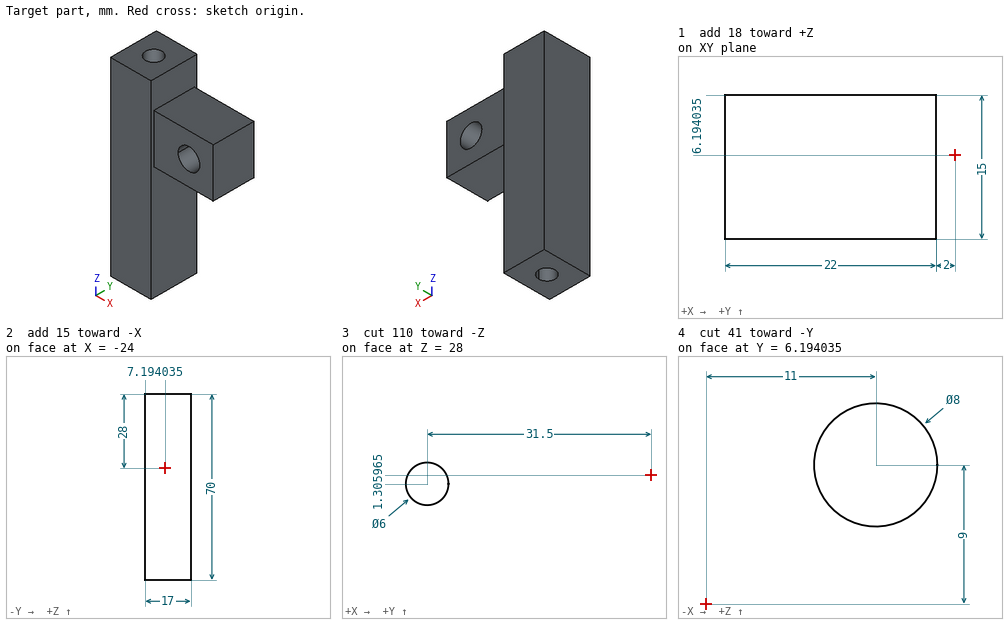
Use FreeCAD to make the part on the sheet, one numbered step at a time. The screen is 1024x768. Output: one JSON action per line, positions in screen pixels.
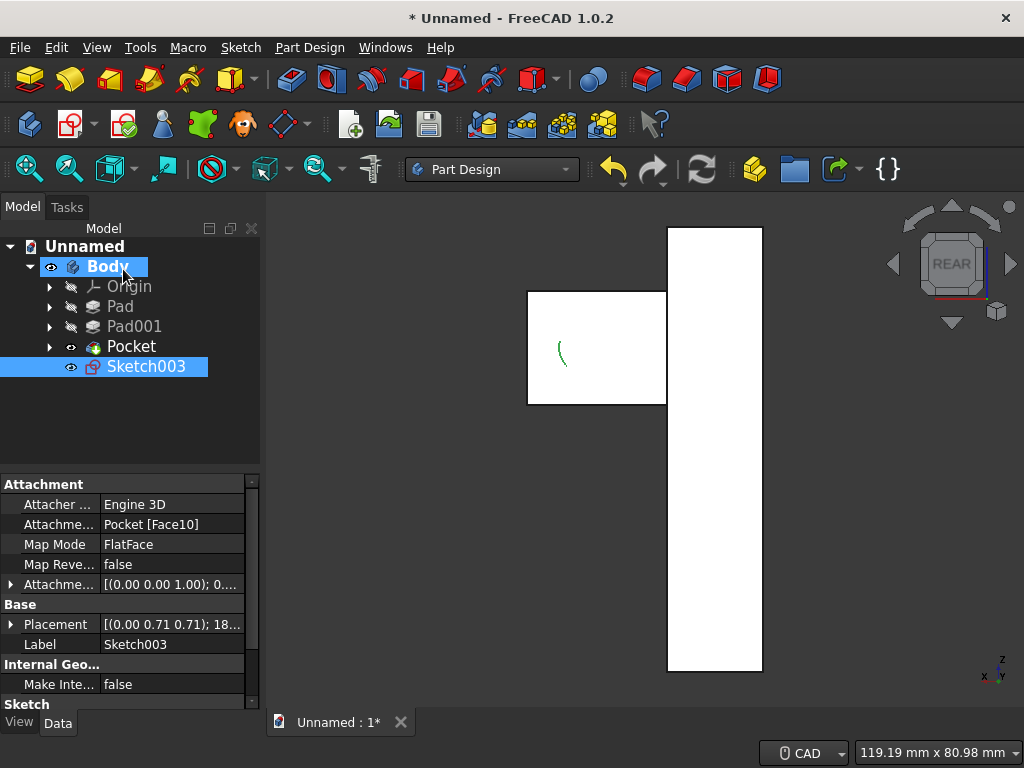
{"action": "left_click", "coordinate": [292, 80]}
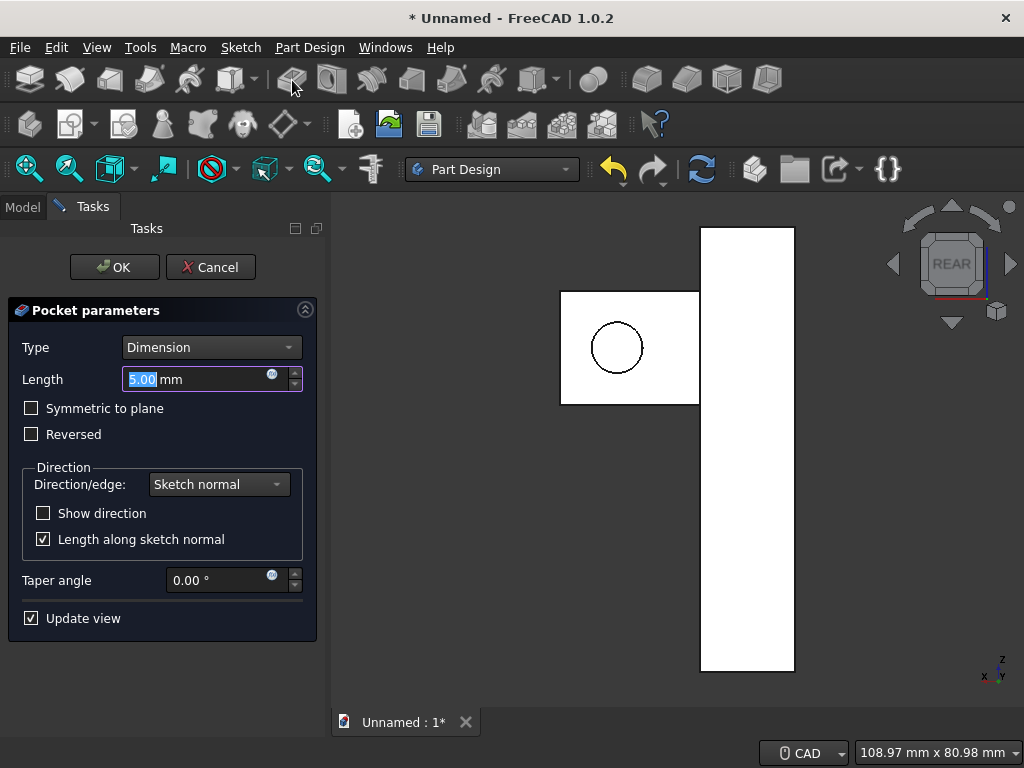
{"action": "type", "text": "41"}
{"action": "key", "text": "Tab"}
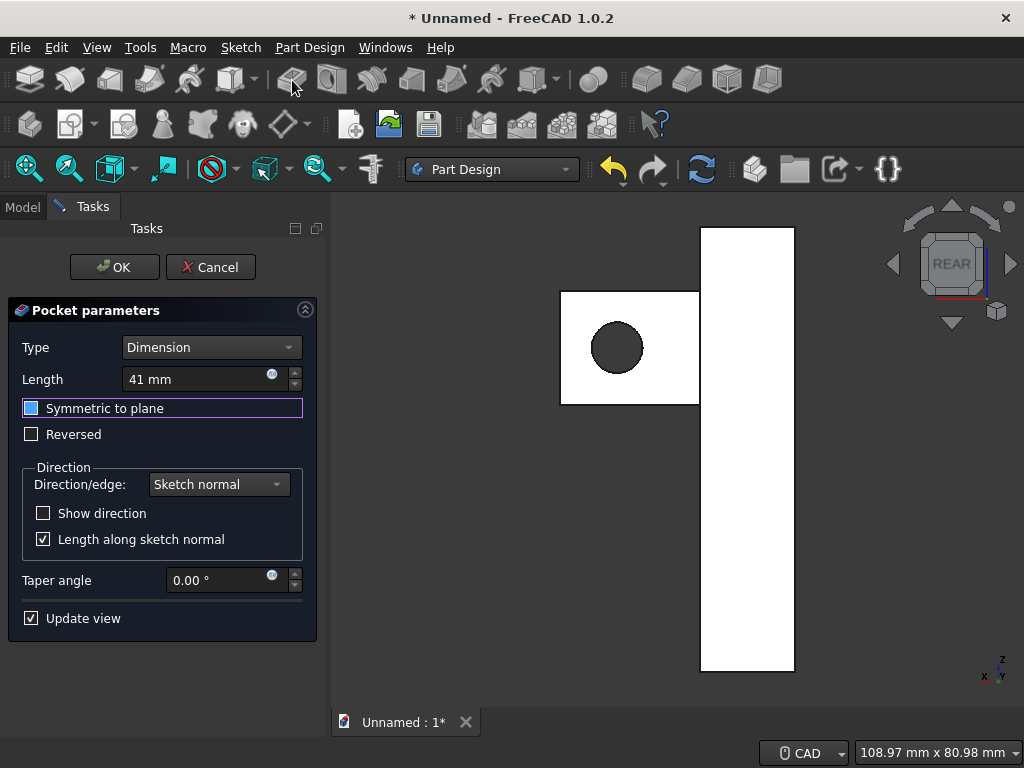
{"action": "left_click", "coordinate": [115, 267]}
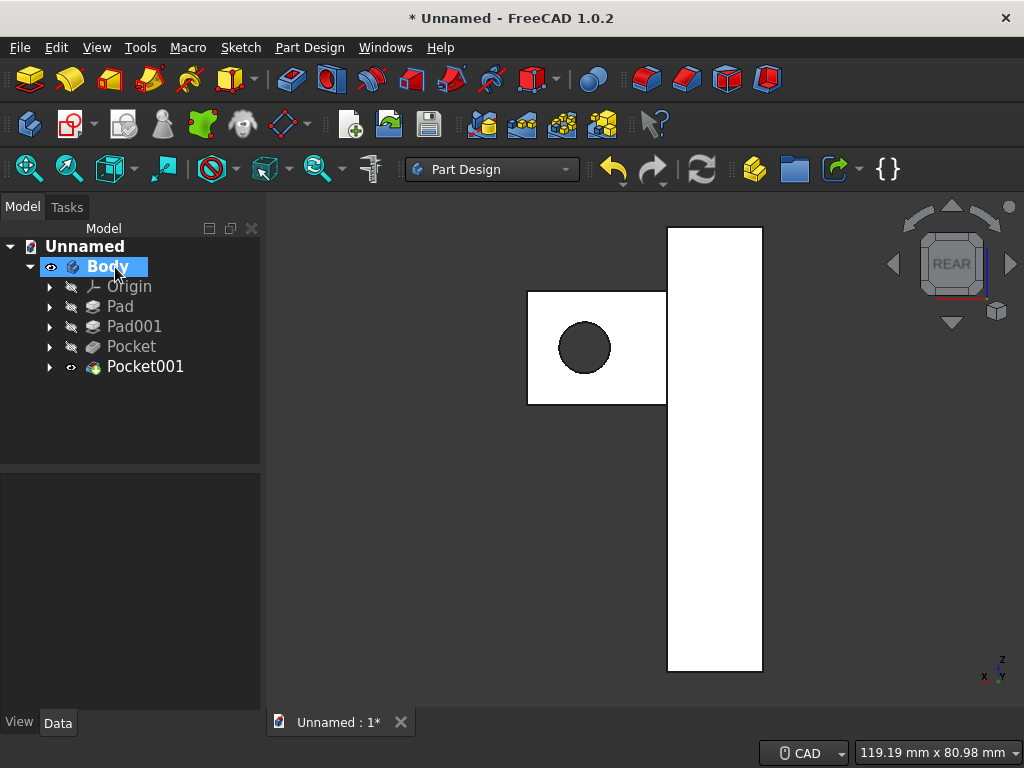
{"action": "key", "text": "0"}